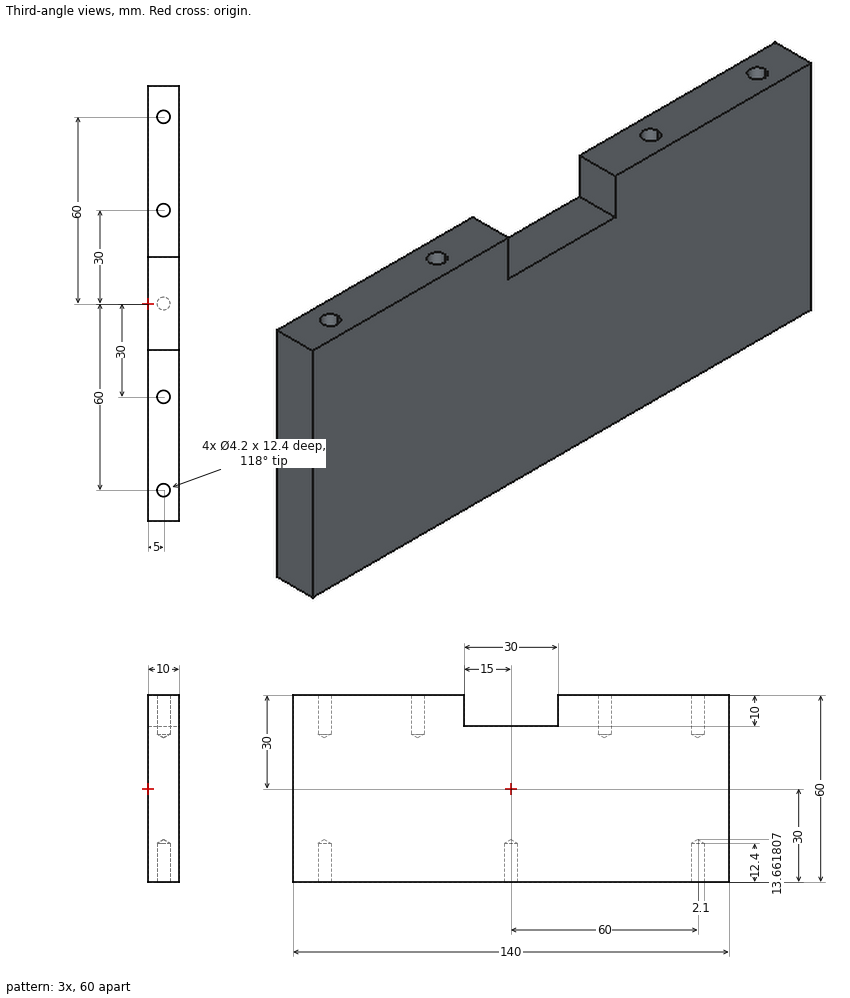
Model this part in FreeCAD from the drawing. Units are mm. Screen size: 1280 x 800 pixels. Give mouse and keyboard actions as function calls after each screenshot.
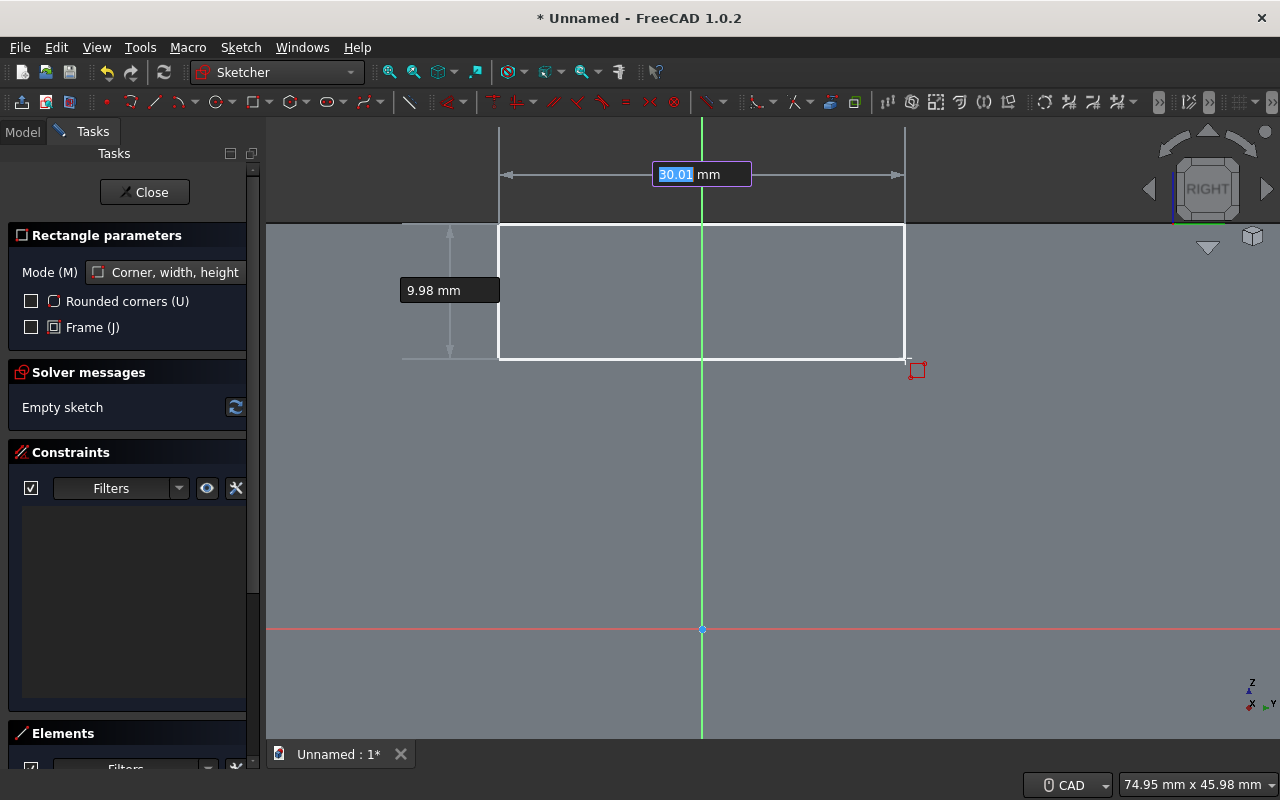
text(30)
key(Tab)
text(10)
key(Return)
key(Escape)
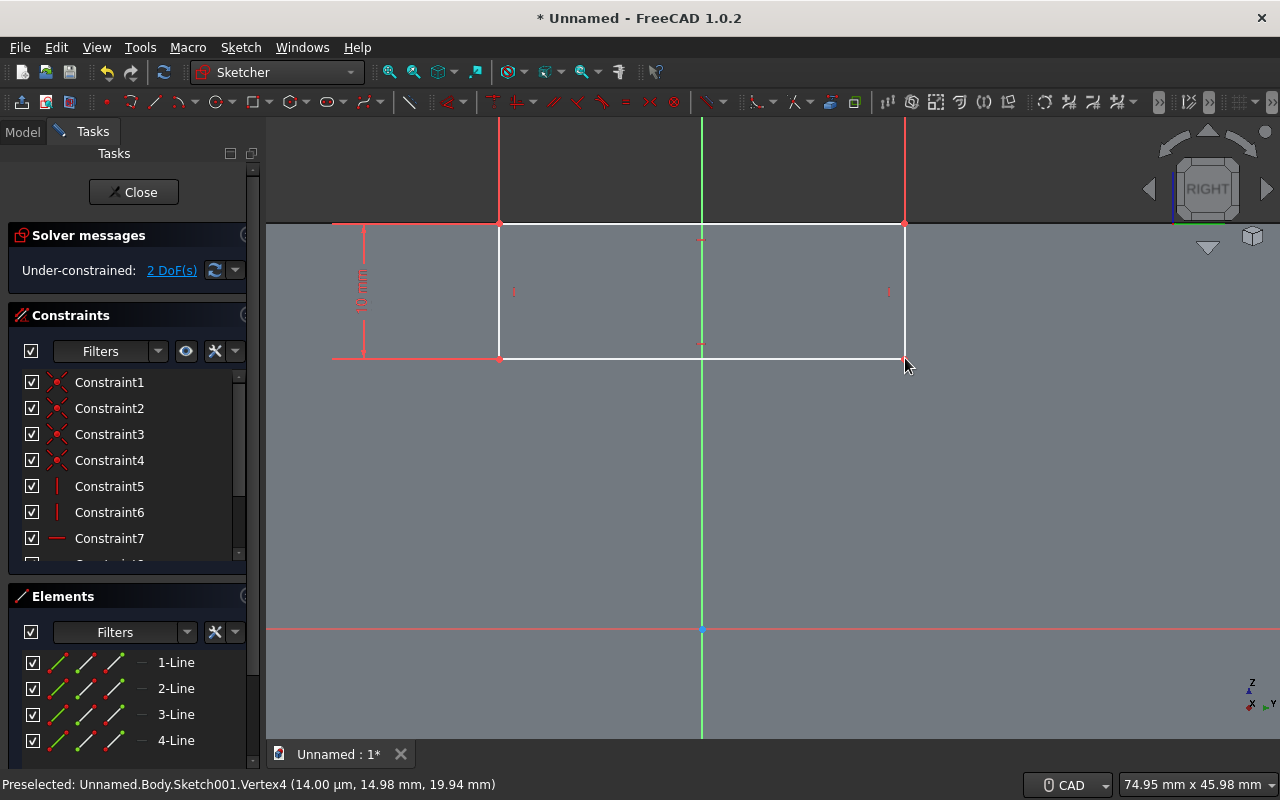
click(448, 102)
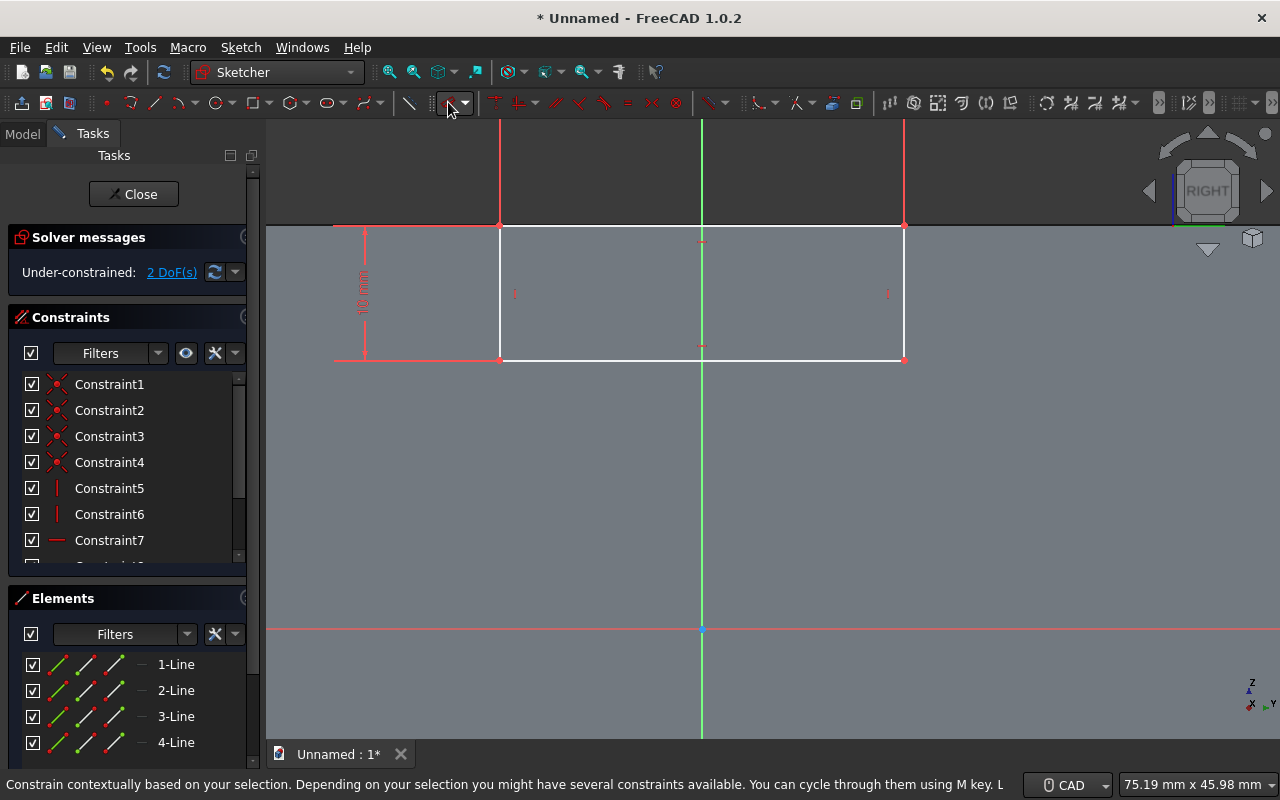
click(500, 226)
click(601, 663)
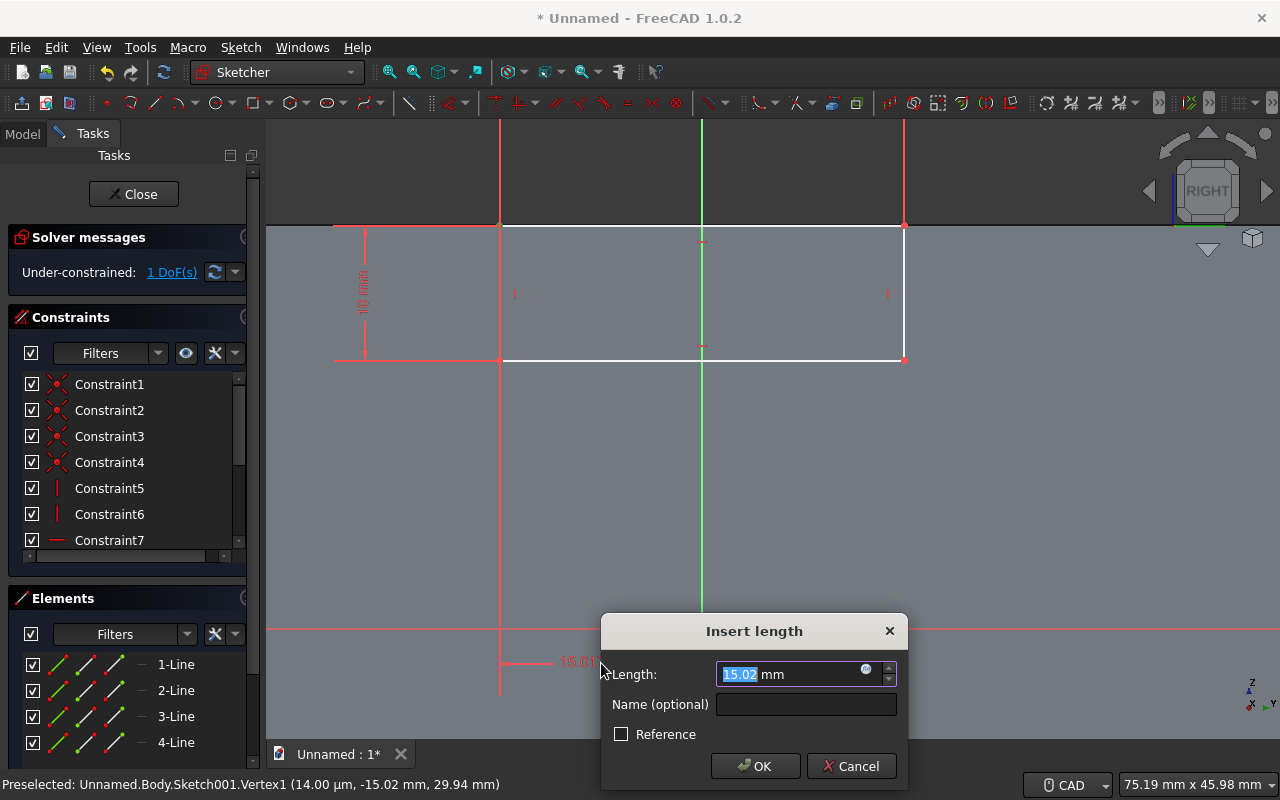
text(15)
key(Return)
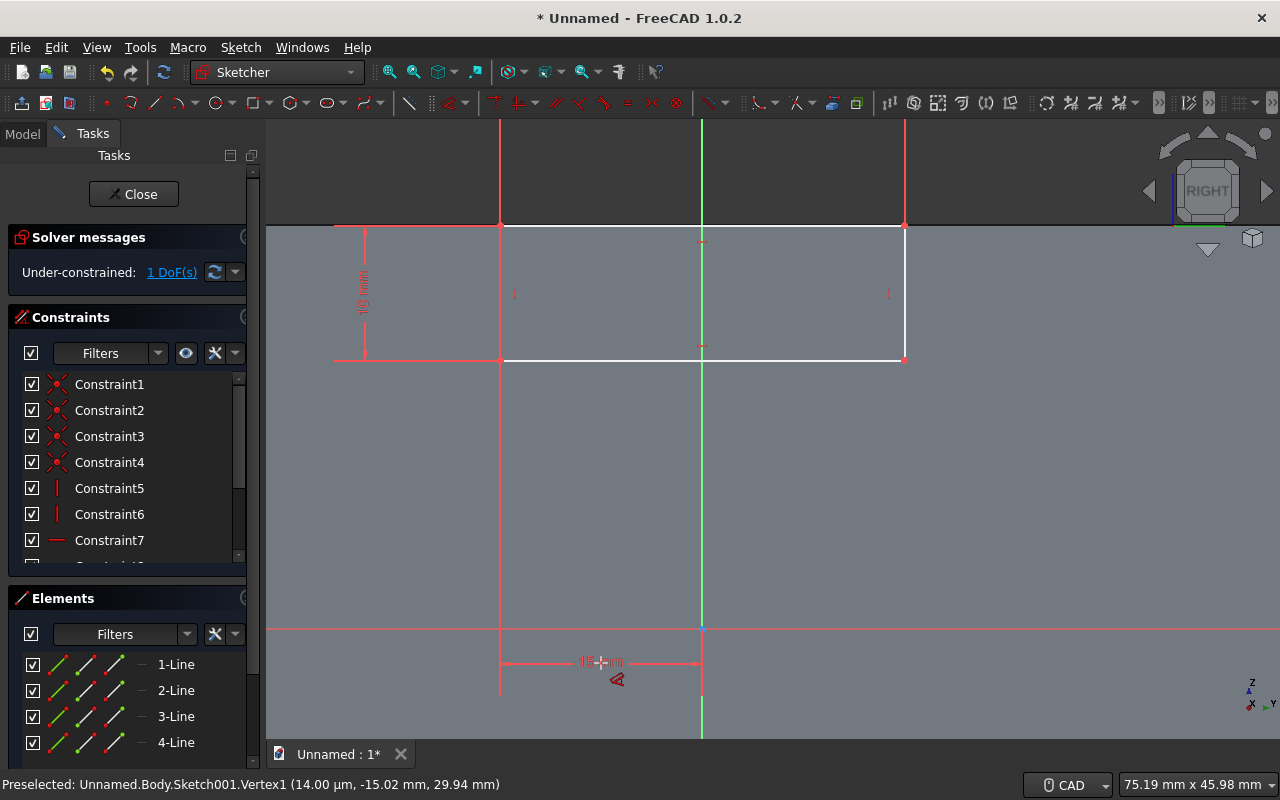
click(500, 226)
click(466, 428)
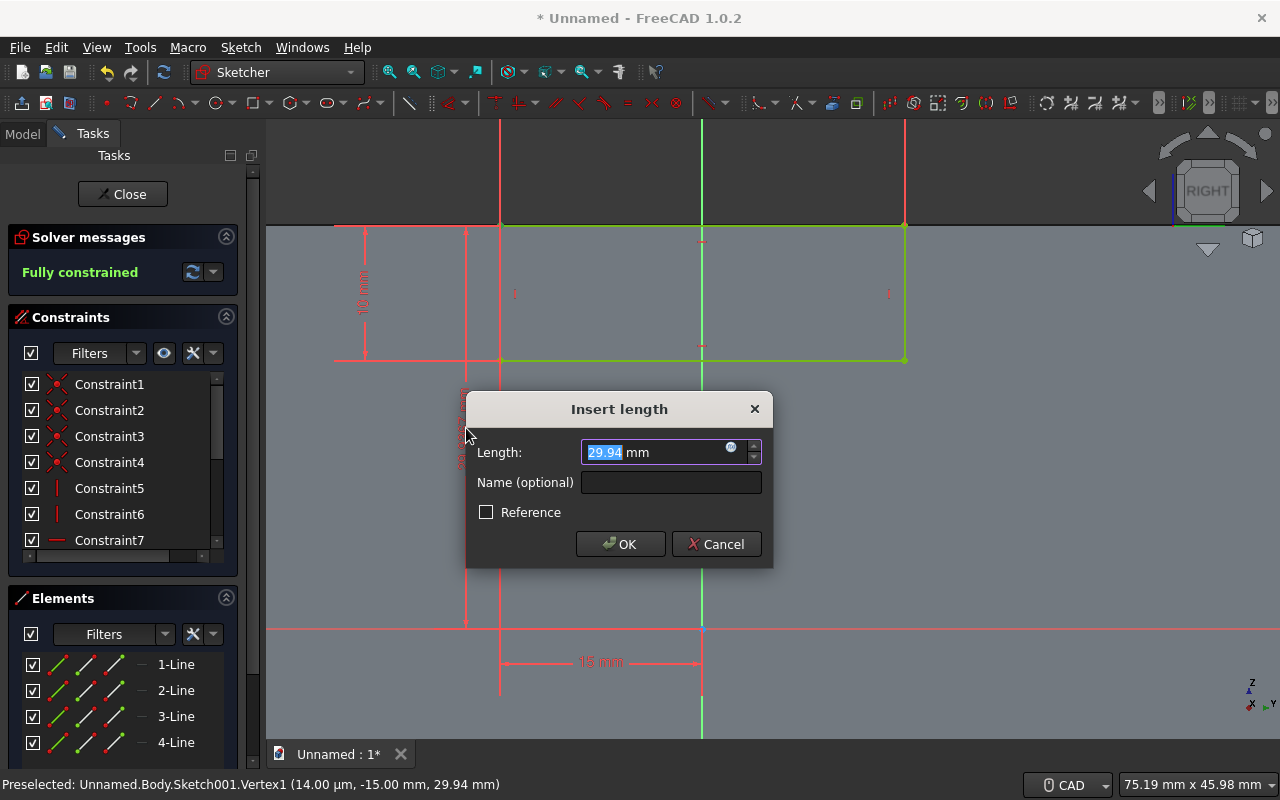
text(30)
key(Return)
key(Escape)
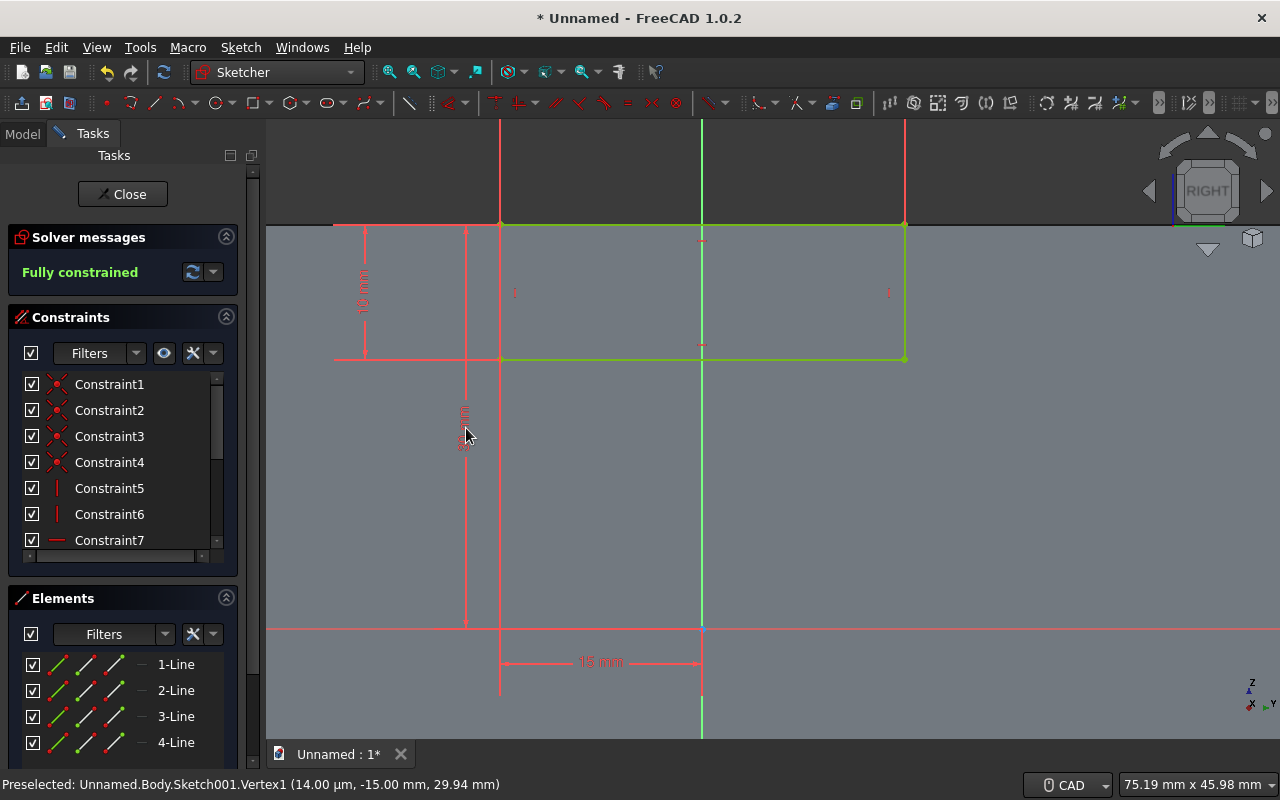
click(123, 194)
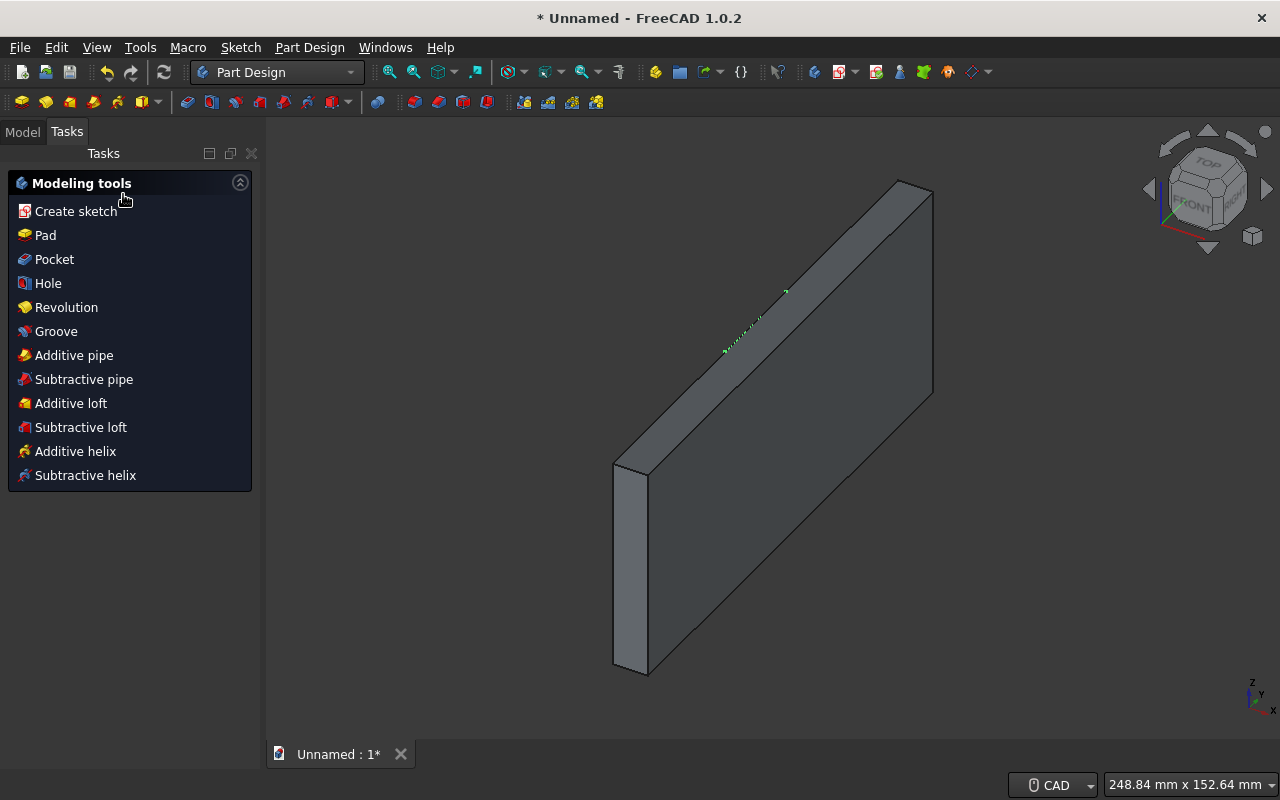
click(188, 102)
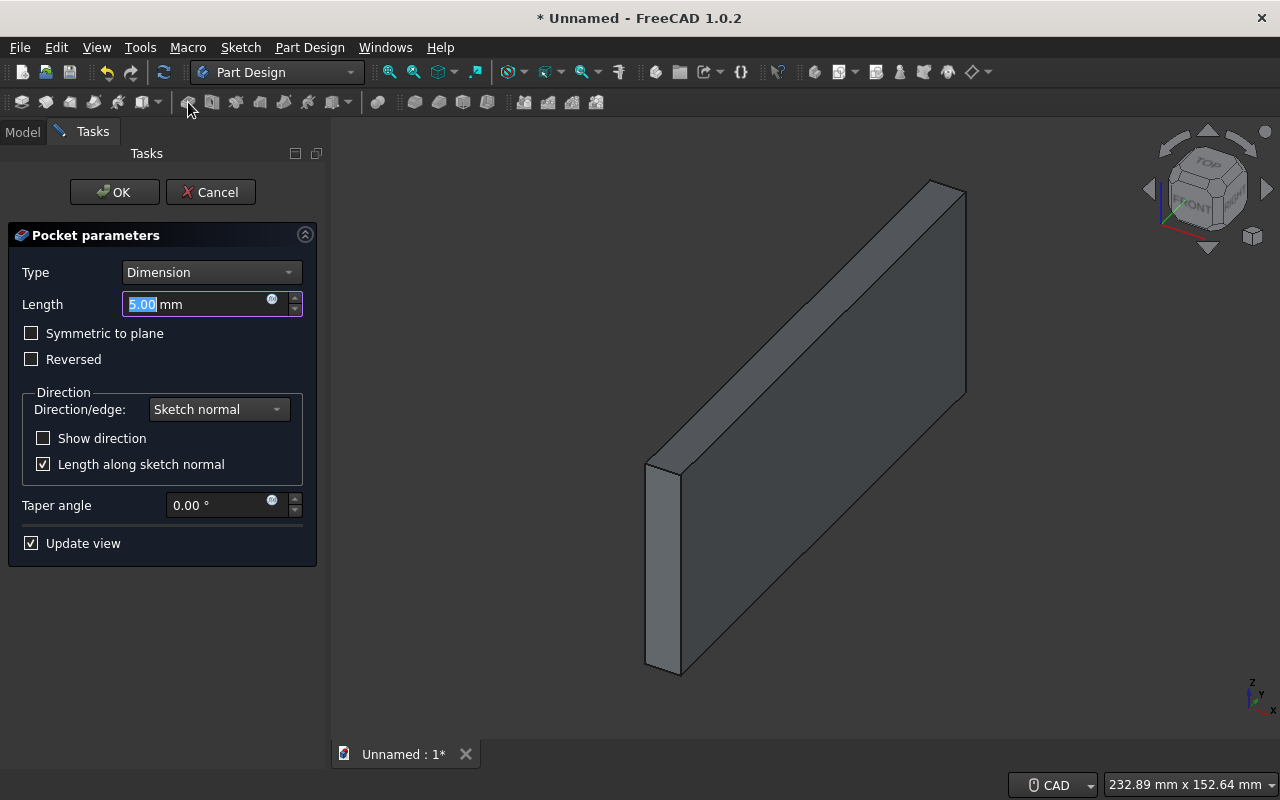
click(212, 272)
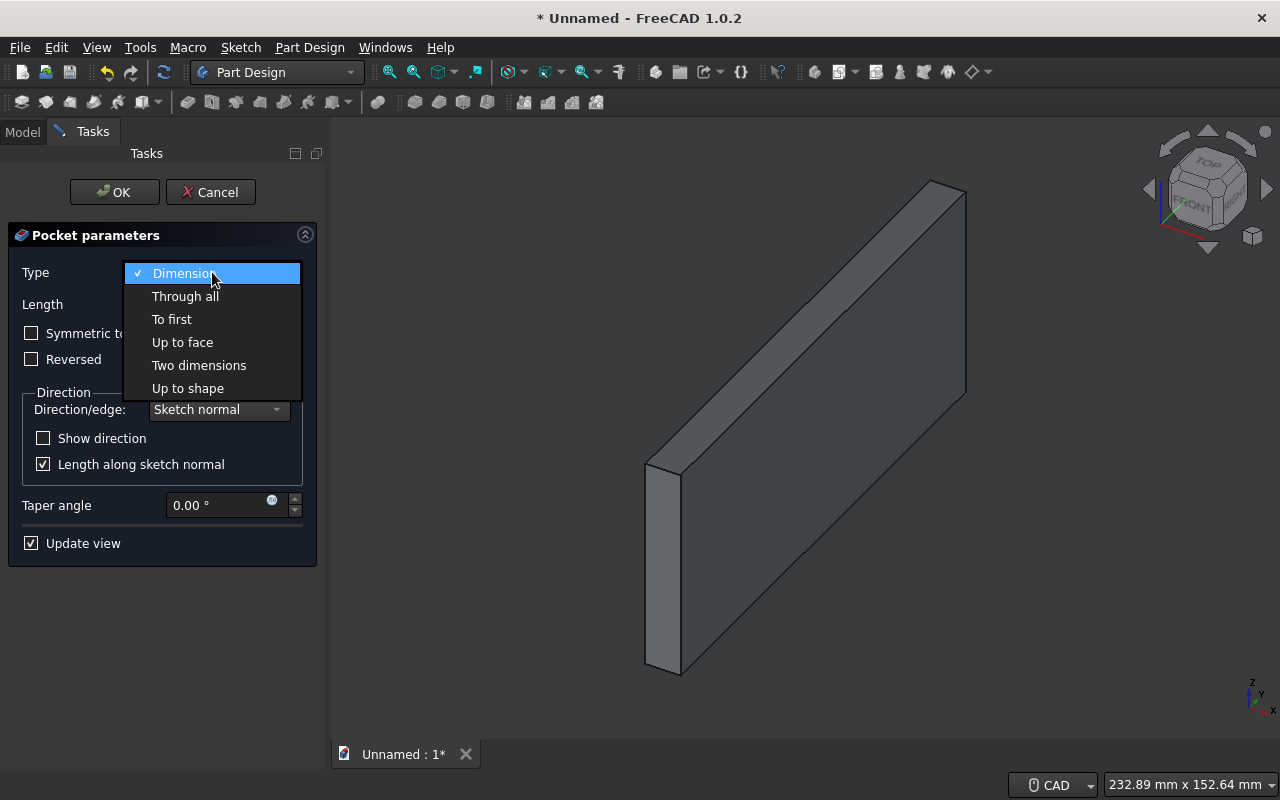
click(212, 296)